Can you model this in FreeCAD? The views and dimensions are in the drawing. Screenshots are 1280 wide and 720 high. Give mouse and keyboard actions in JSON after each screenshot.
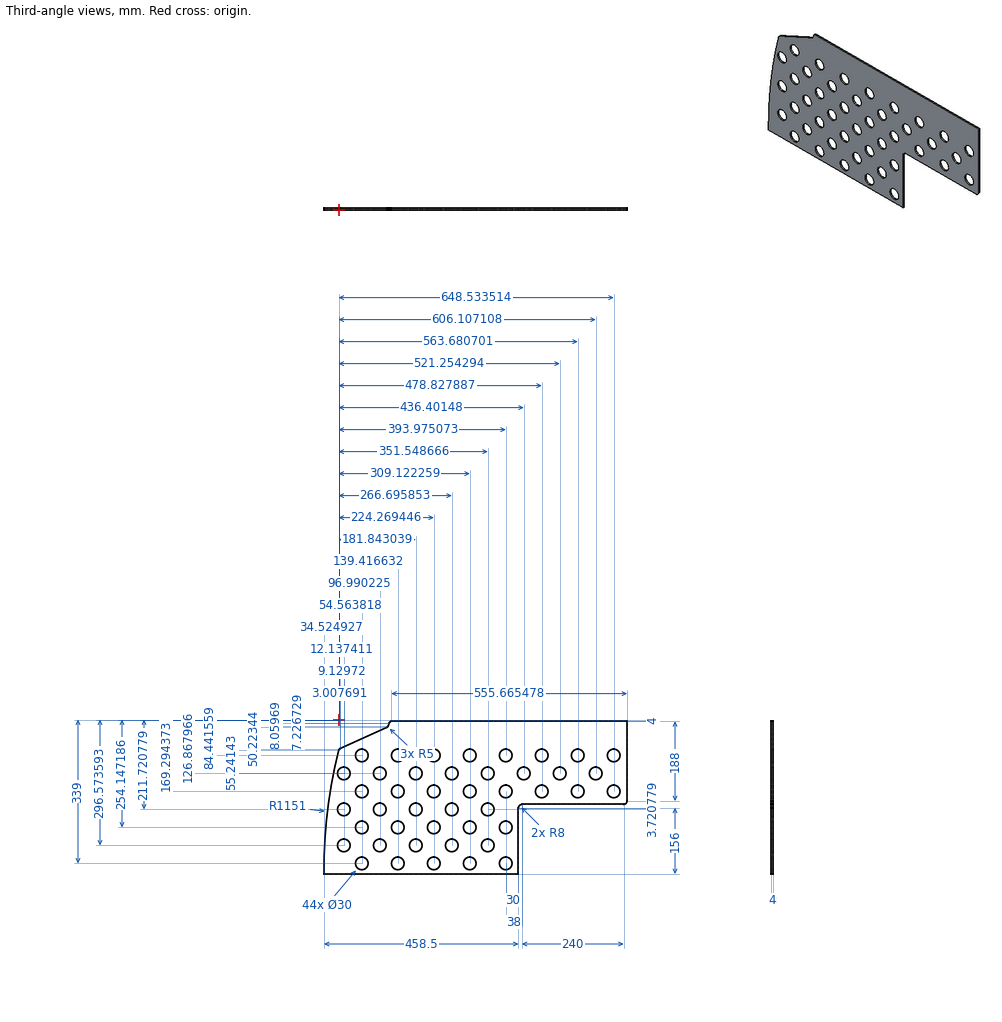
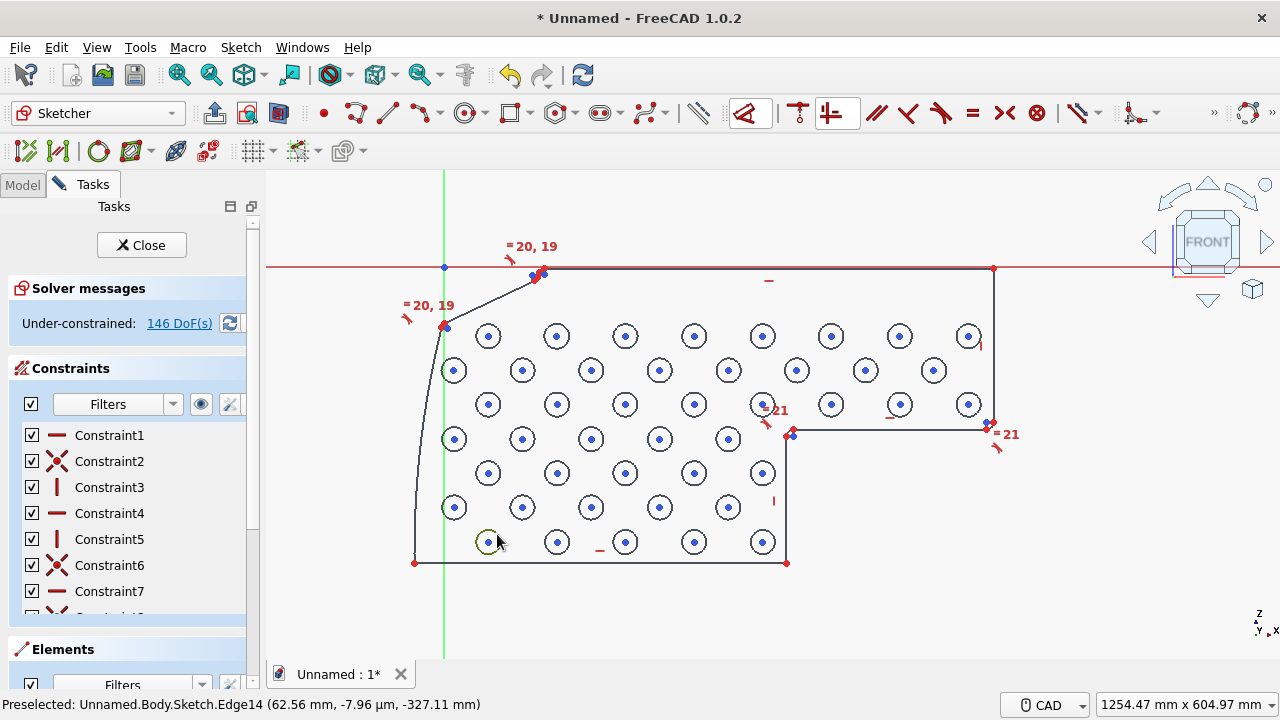
{"action": "left_click", "coordinate": [566, 534]}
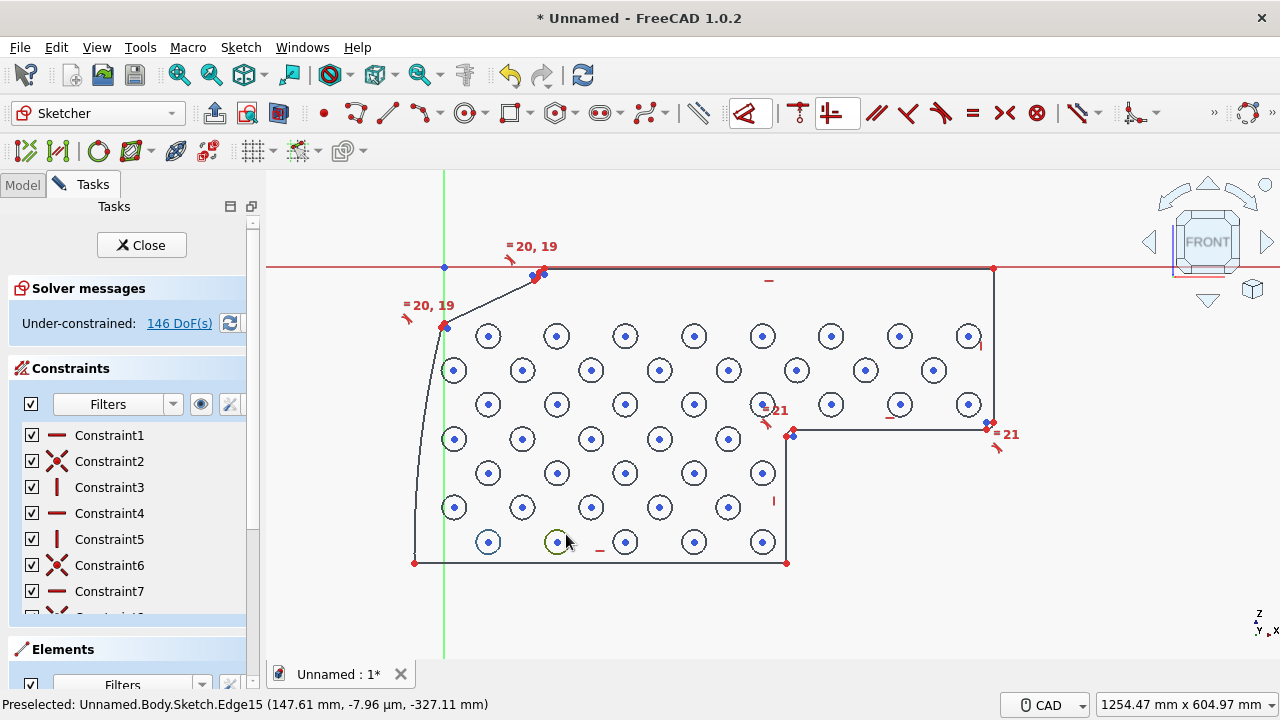
{"action": "left_click", "coordinate": [463, 499]}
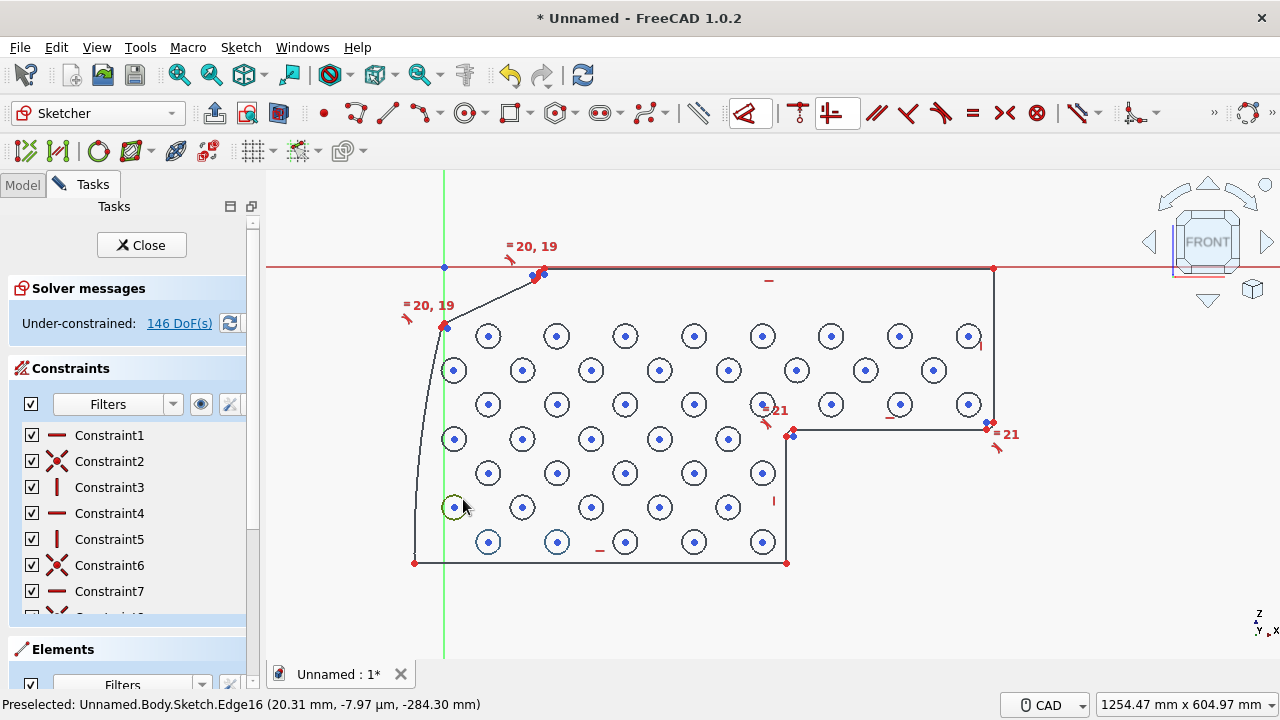
{"action": "left_click", "coordinate": [531, 499]}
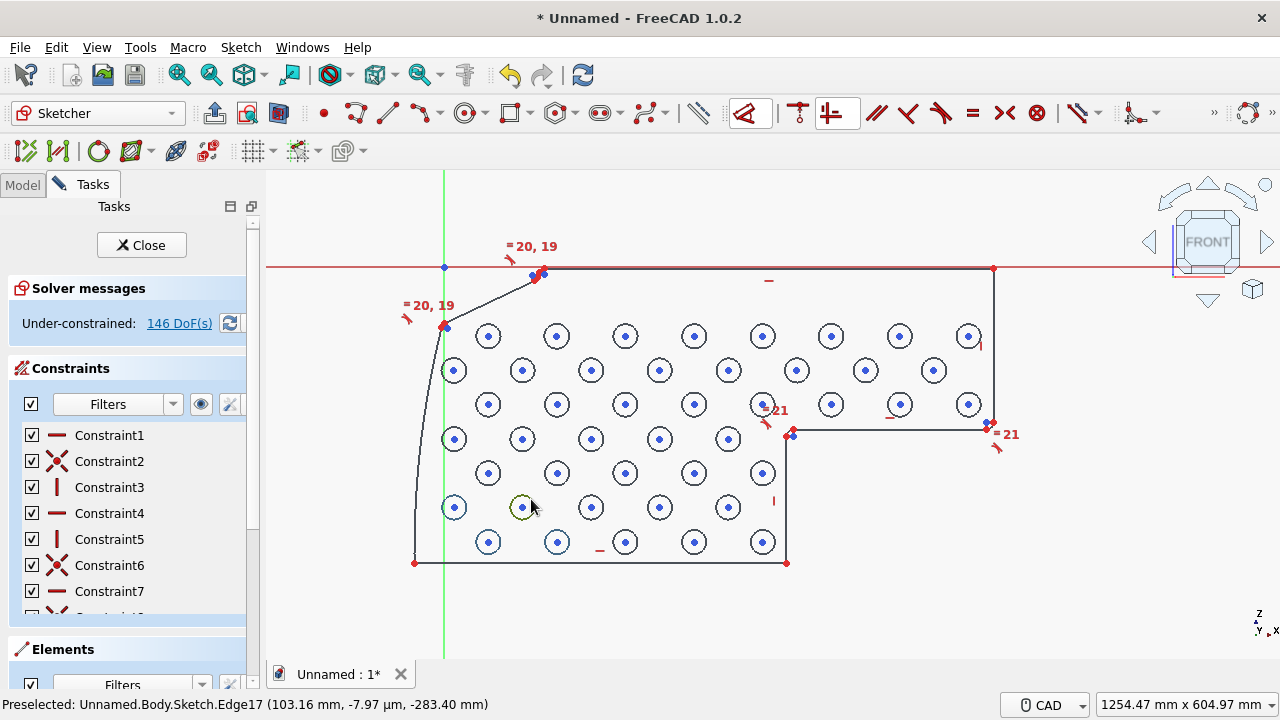
{"action": "left_click", "coordinate": [634, 534]}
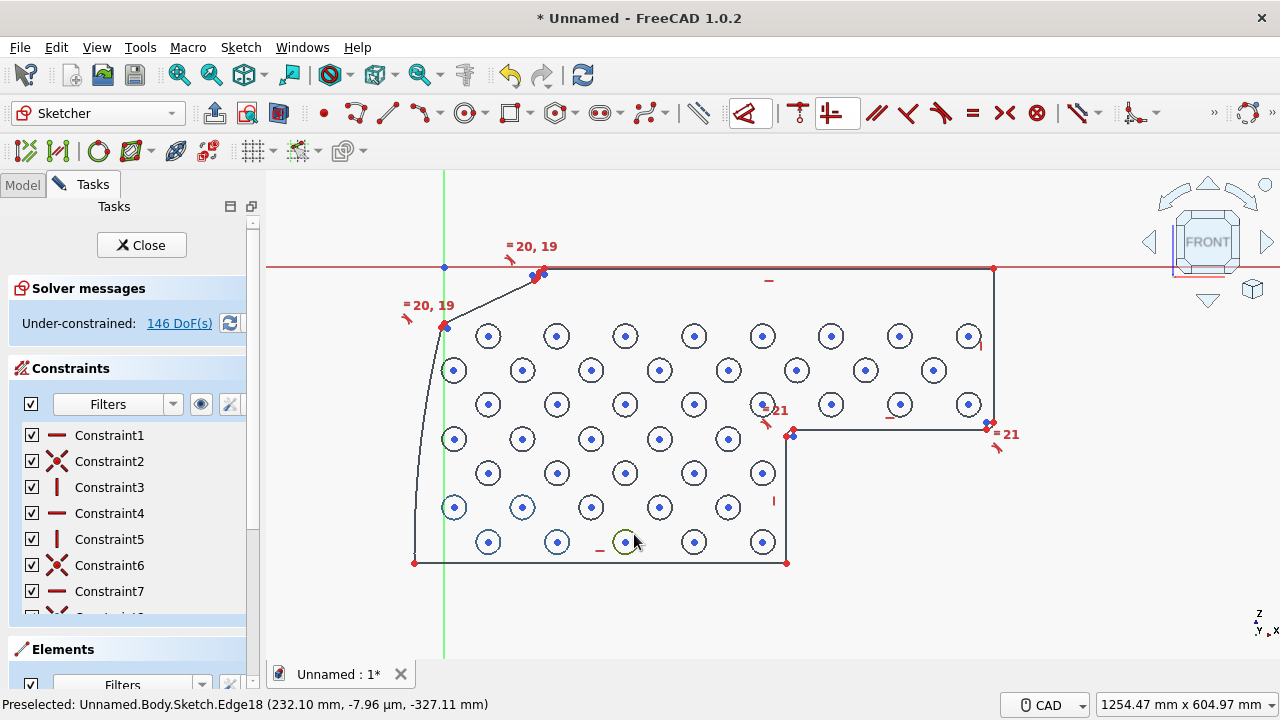
{"action": "left_click", "coordinate": [703, 534]}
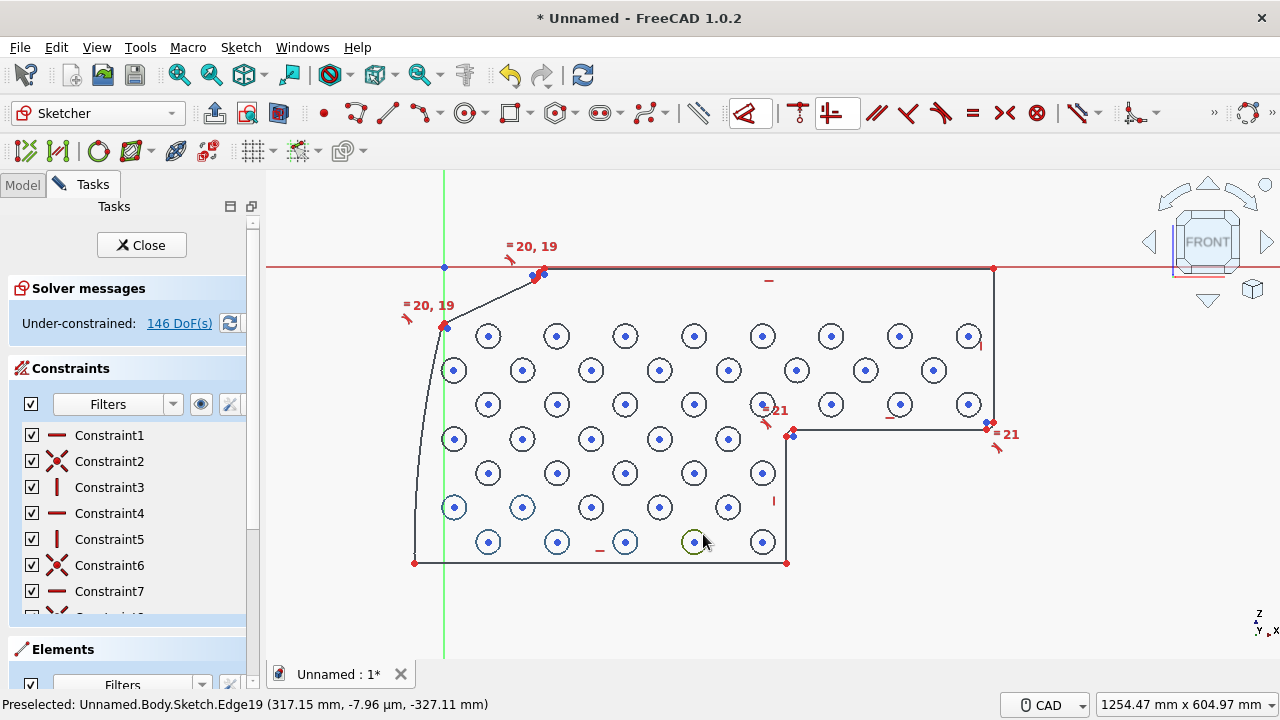
{"action": "left_click", "coordinate": [600, 499]}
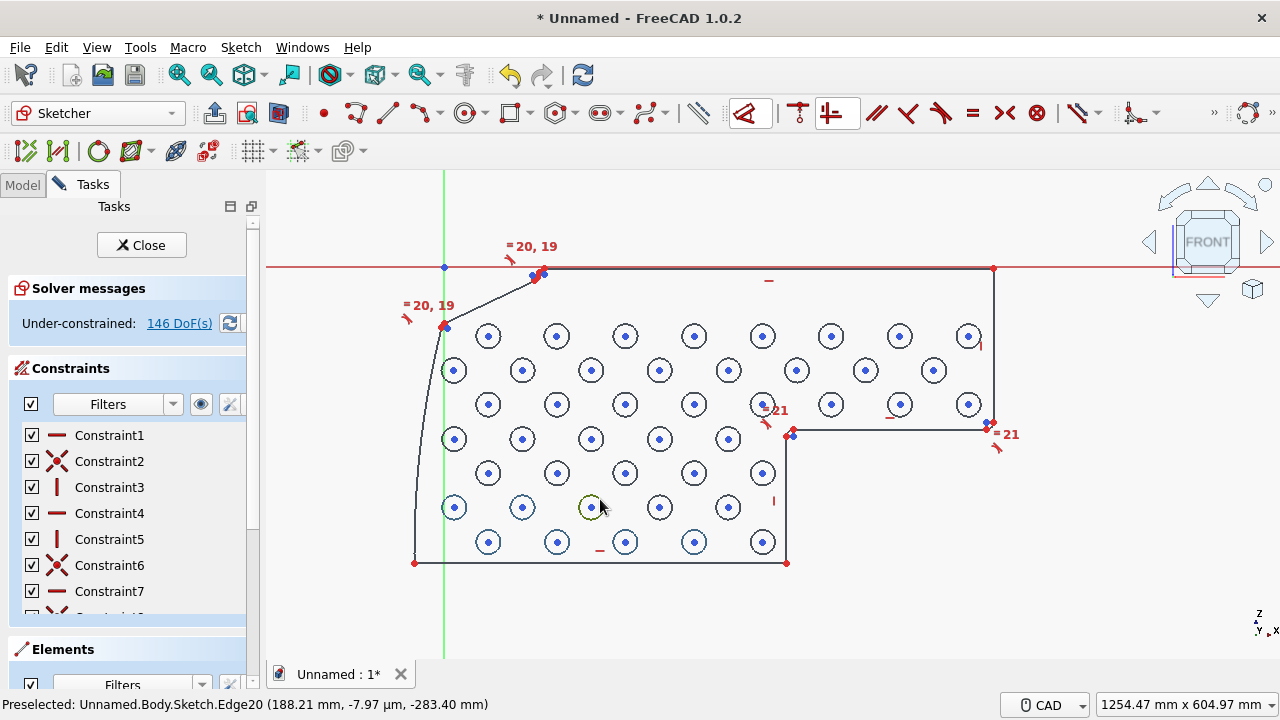
{"action": "left_click", "coordinate": [669, 499]}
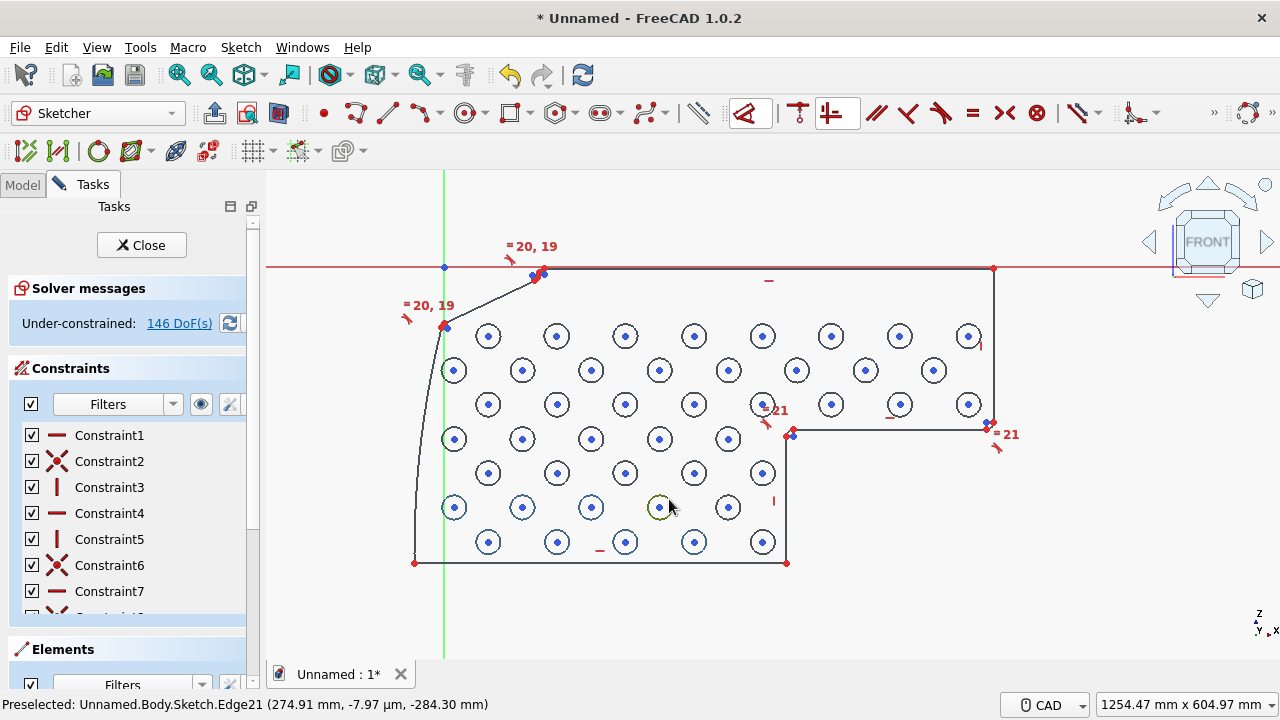
{"action": "left_click", "coordinate": [497, 465]}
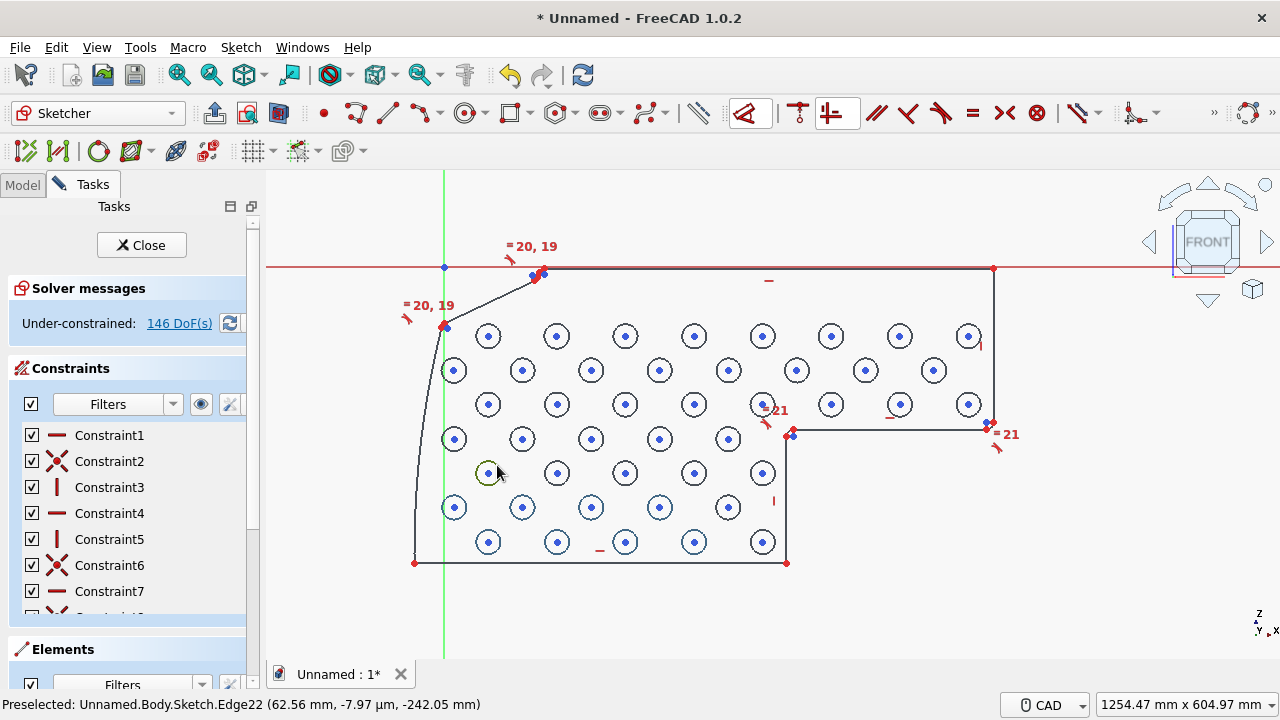
{"action": "left_click", "coordinate": [566, 465]}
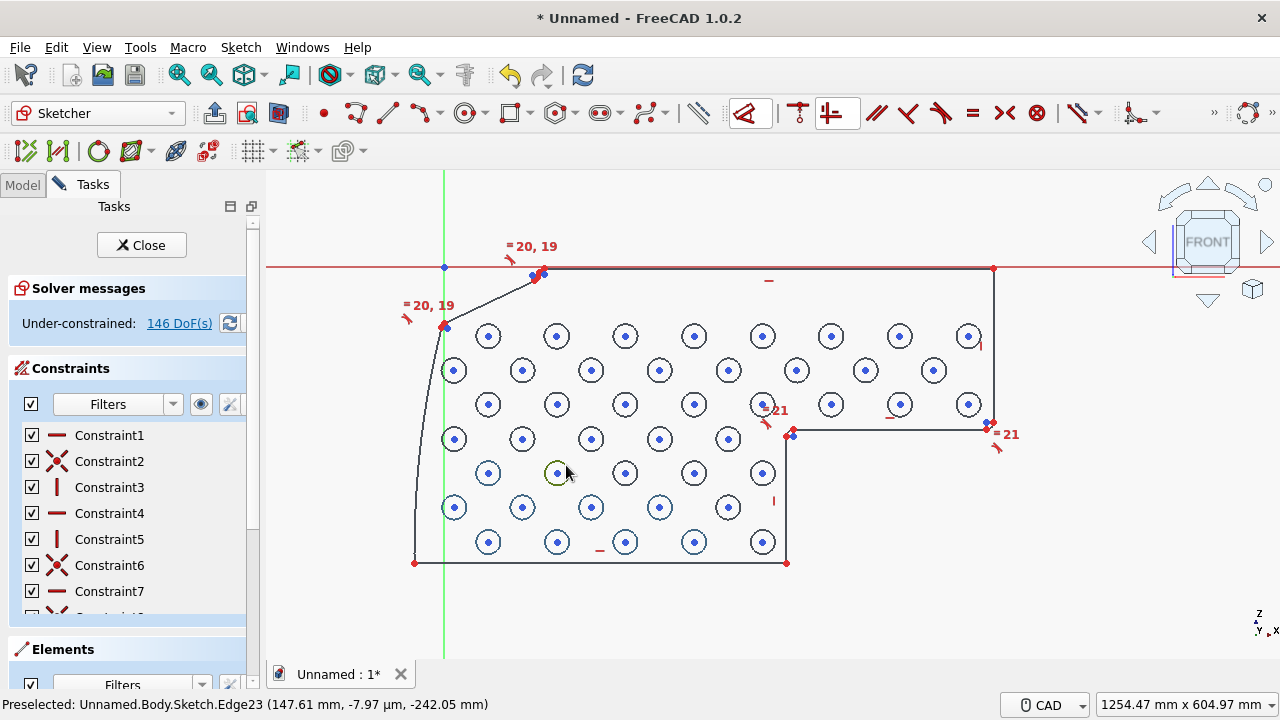
{"action": "left_click", "coordinate": [634, 465]}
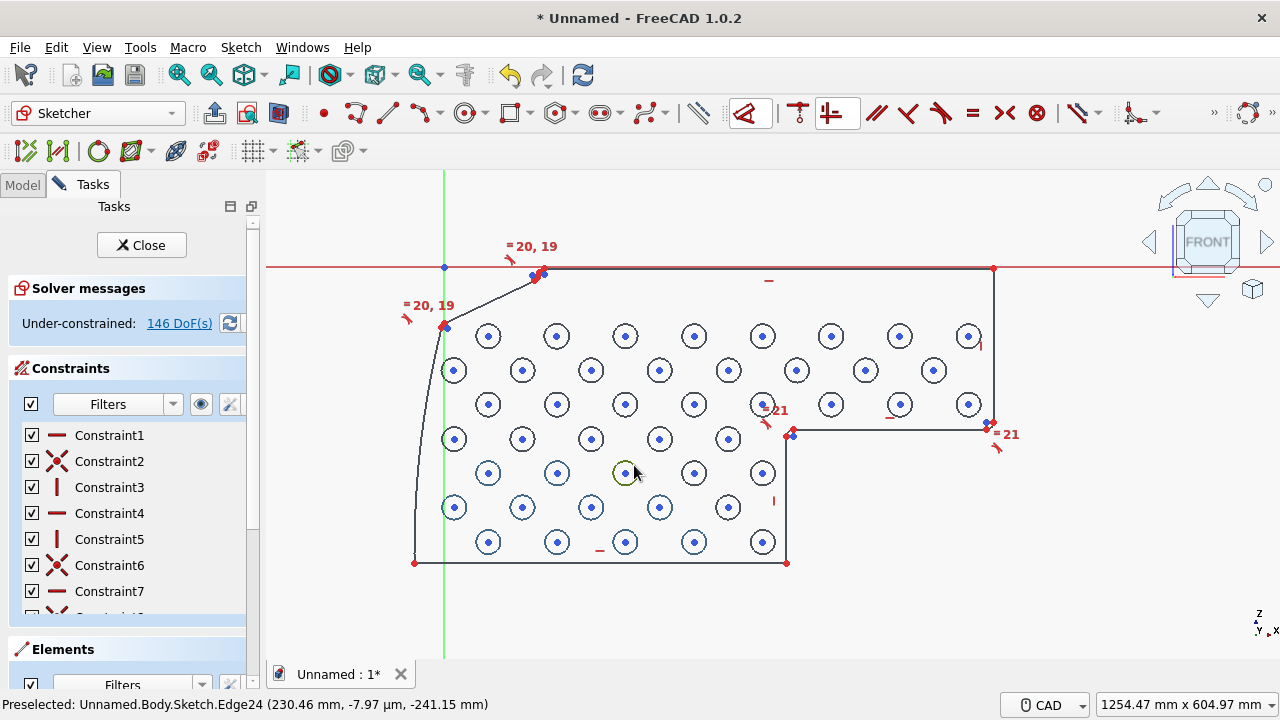
{"action": "left_click", "coordinate": [703, 465]}